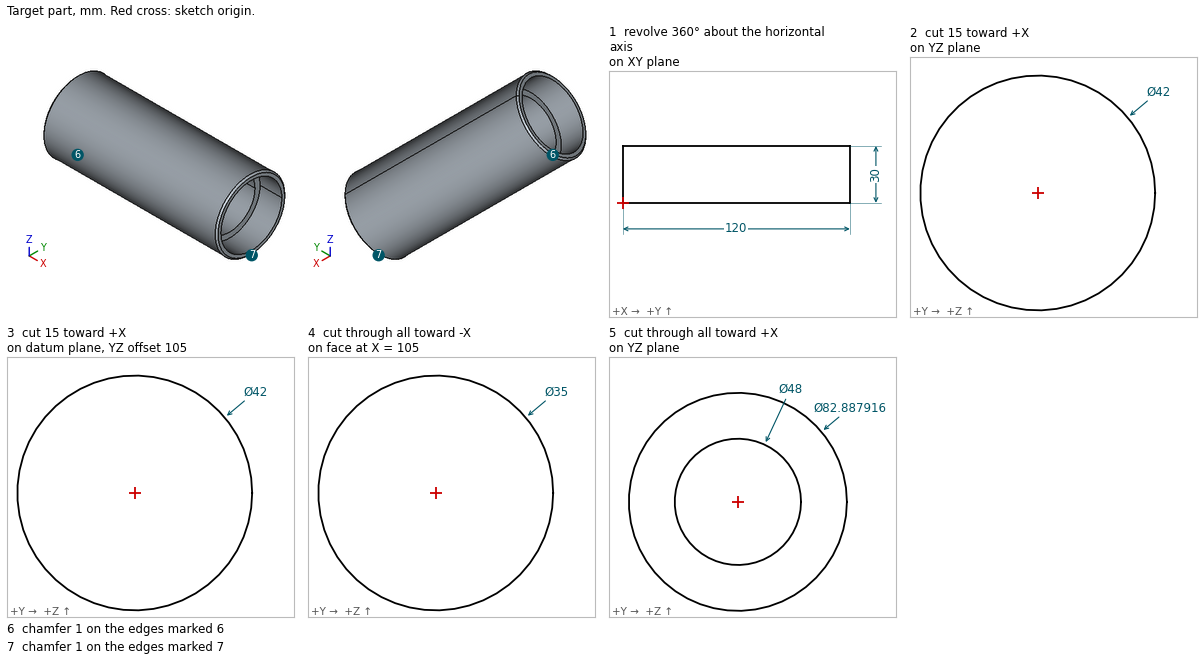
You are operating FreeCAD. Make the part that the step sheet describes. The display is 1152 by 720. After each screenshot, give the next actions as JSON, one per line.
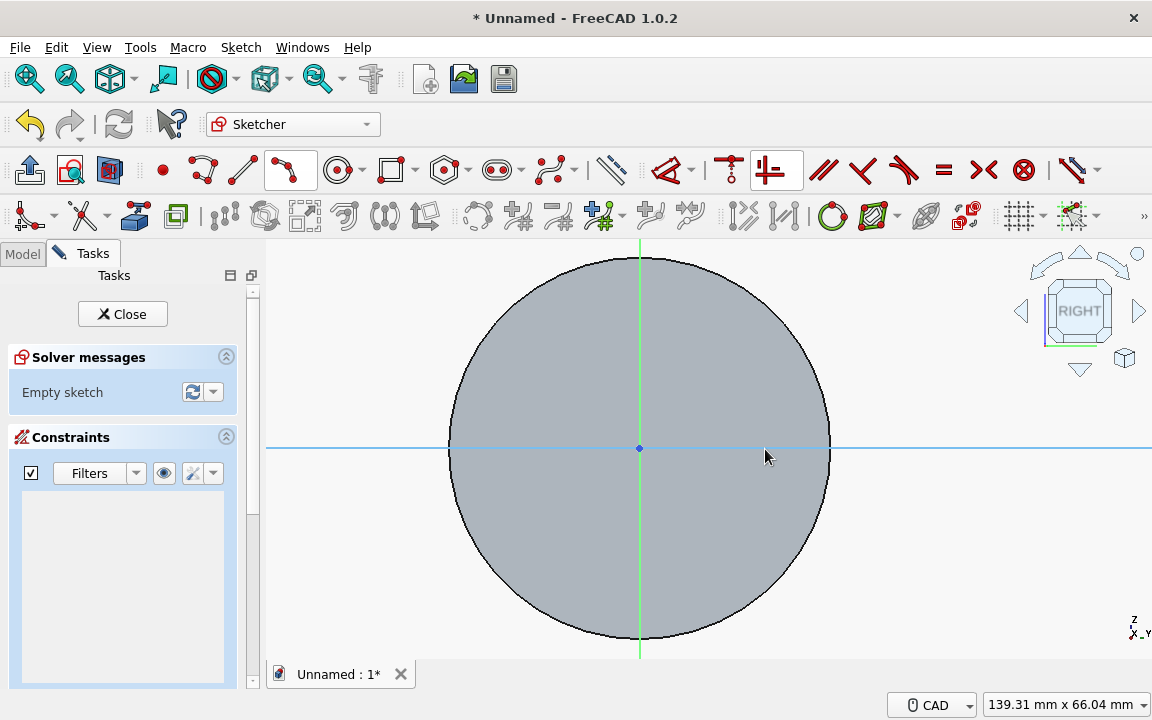
{"action": "key", "text": "g c"}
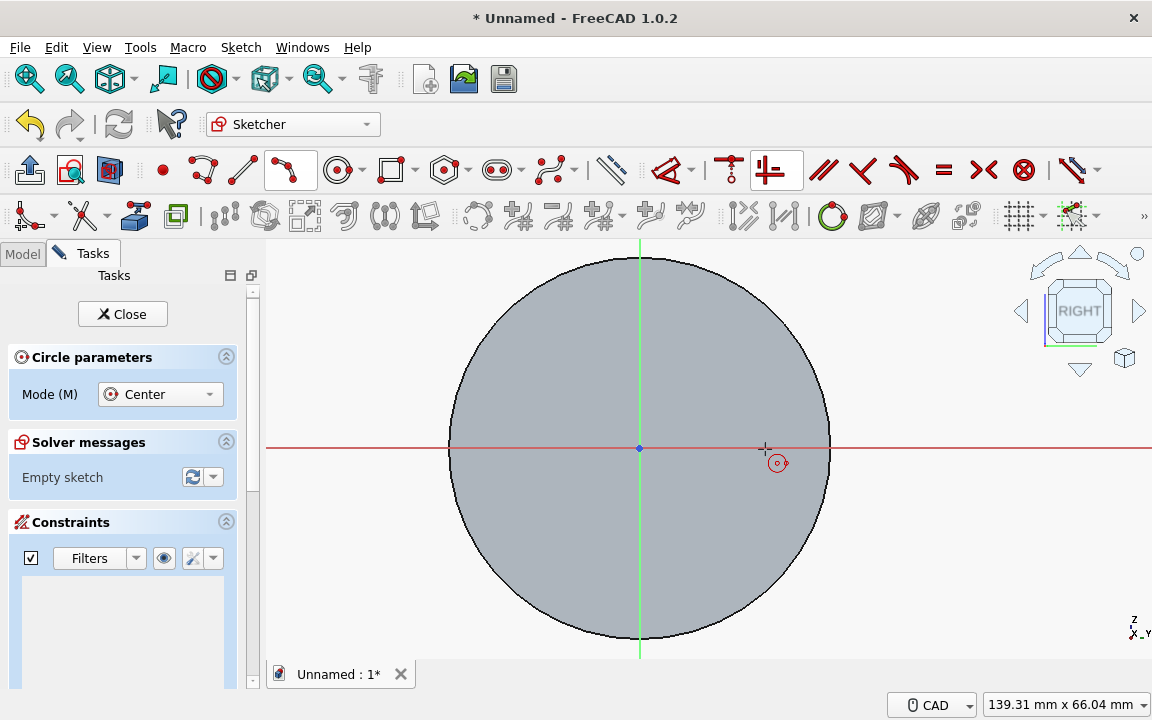
{"action": "left_click", "coordinate": [640, 448]}
{"action": "left_click", "coordinate": [734, 354]}
{"action": "key", "text": "Escape"}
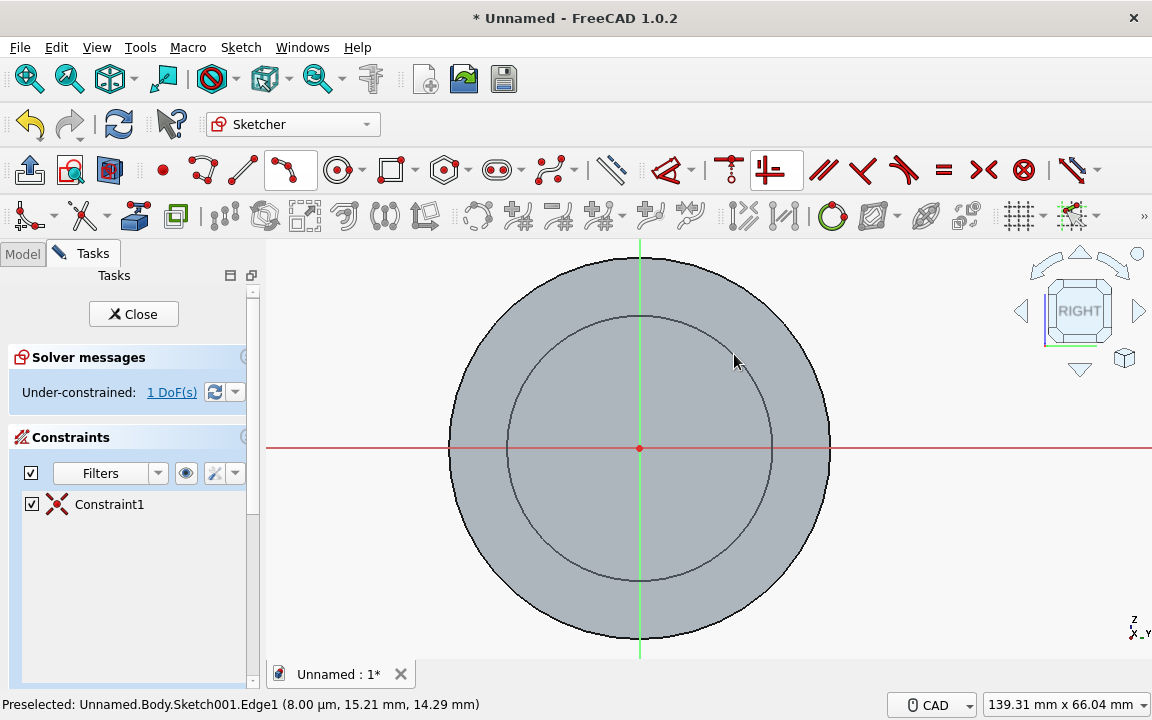
{"action": "left_click", "coordinate": [666, 170]}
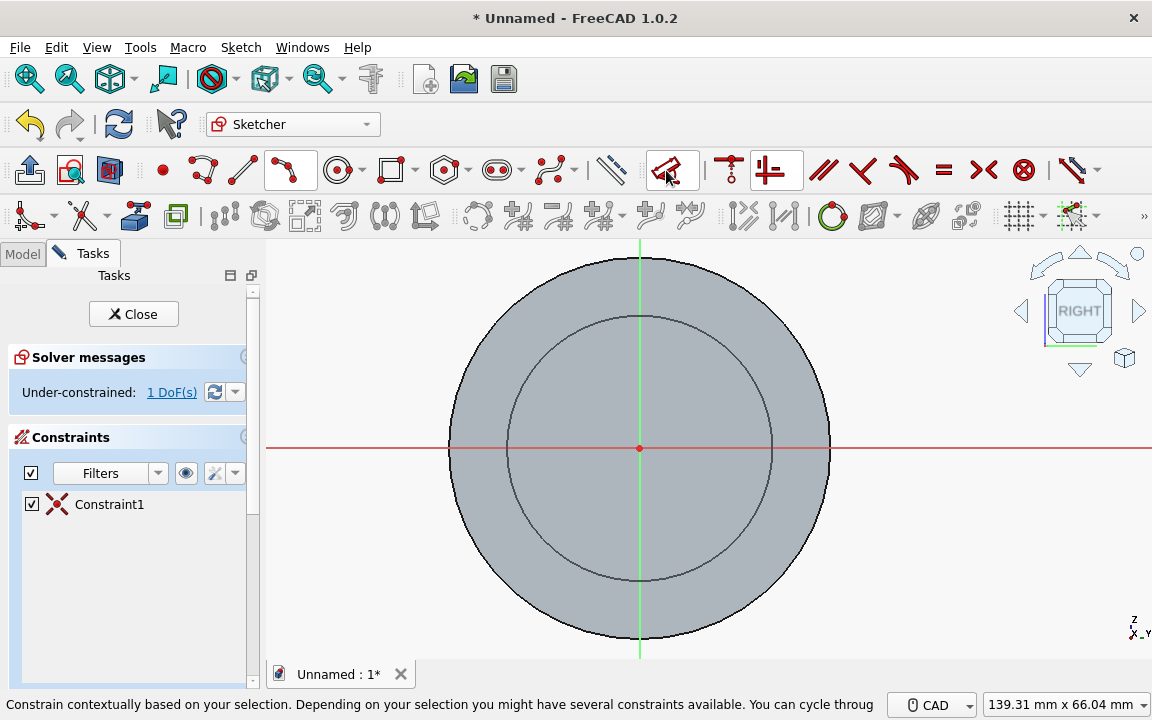
{"action": "left_click", "coordinate": [733, 354]}
{"action": "left_click", "coordinate": [755, 331]}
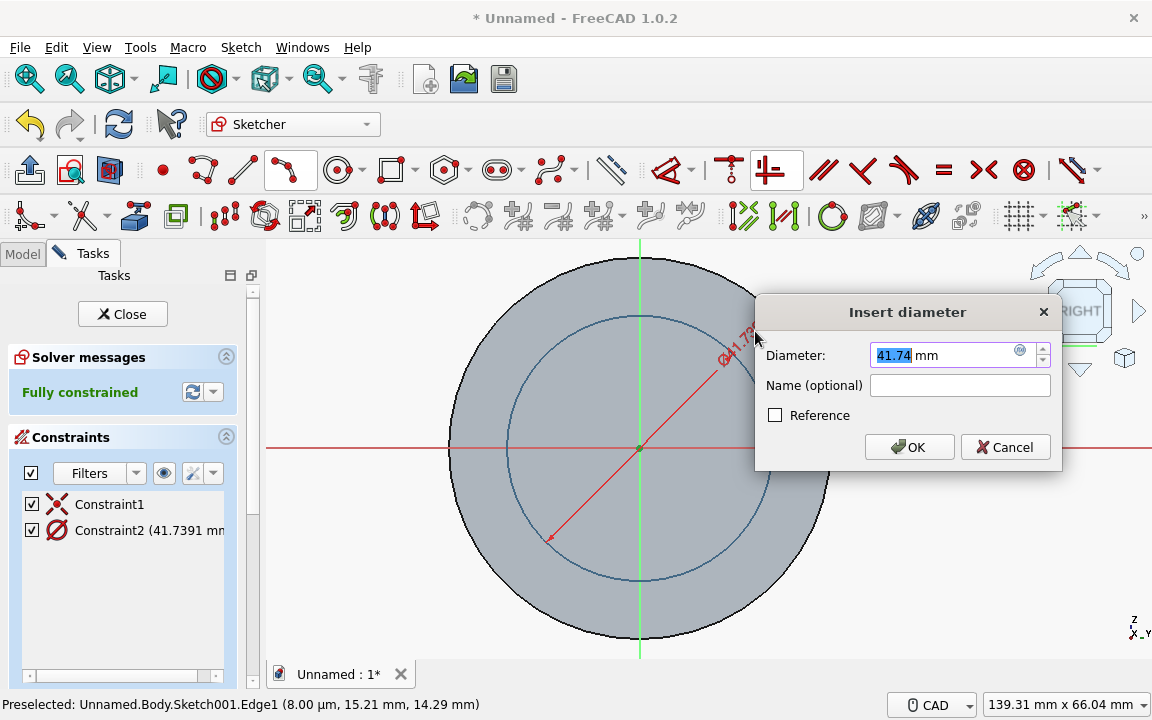
{"action": "type", "text": "42"}
{"action": "key", "text": "Return"}
{"action": "key", "text": "Escape"}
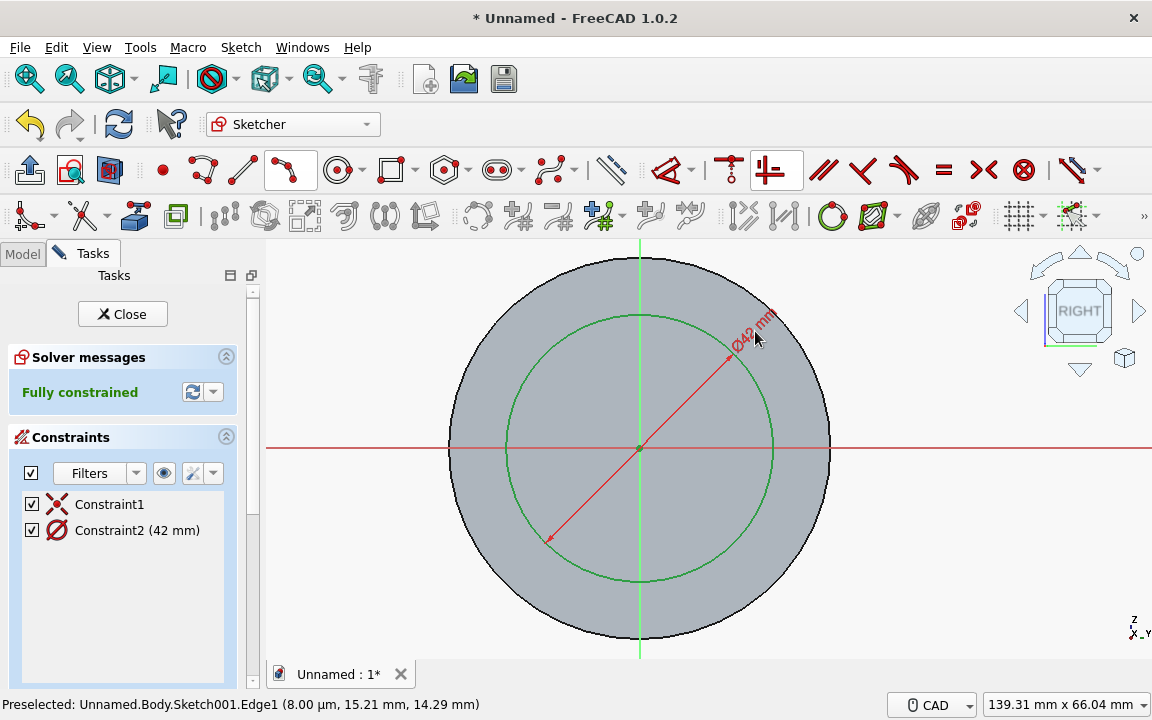
{"action": "left_click", "coordinate": [123, 314]}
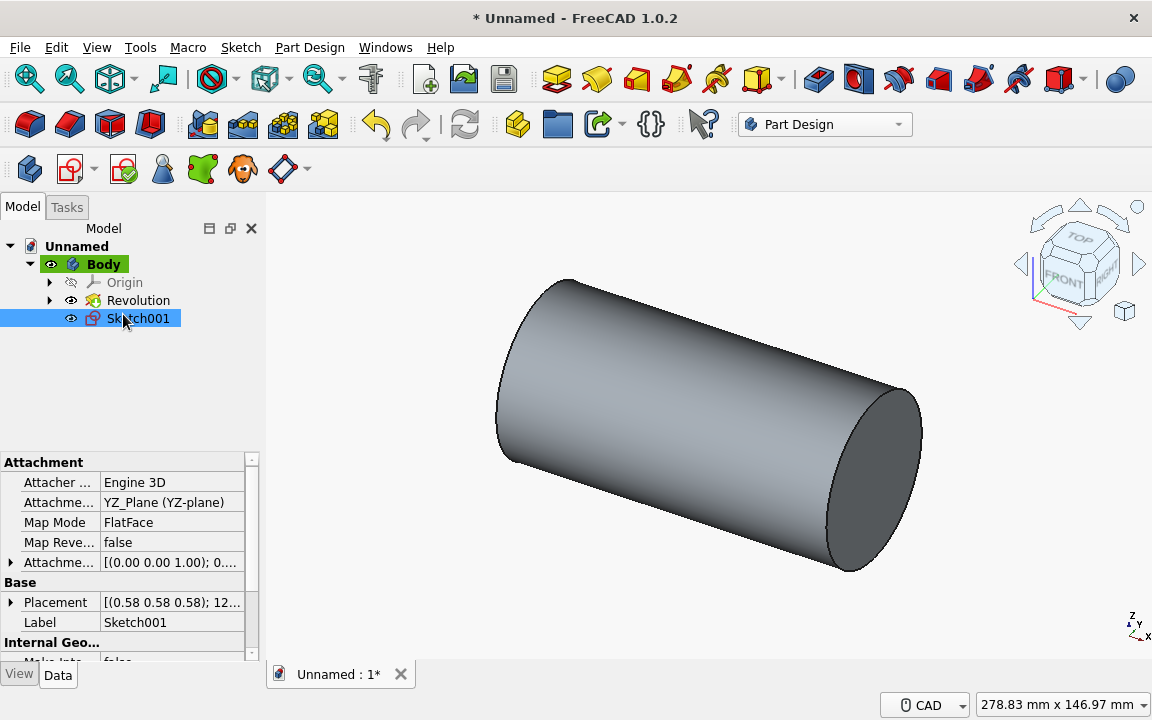
{"action": "left_click", "coordinate": [820, 80]}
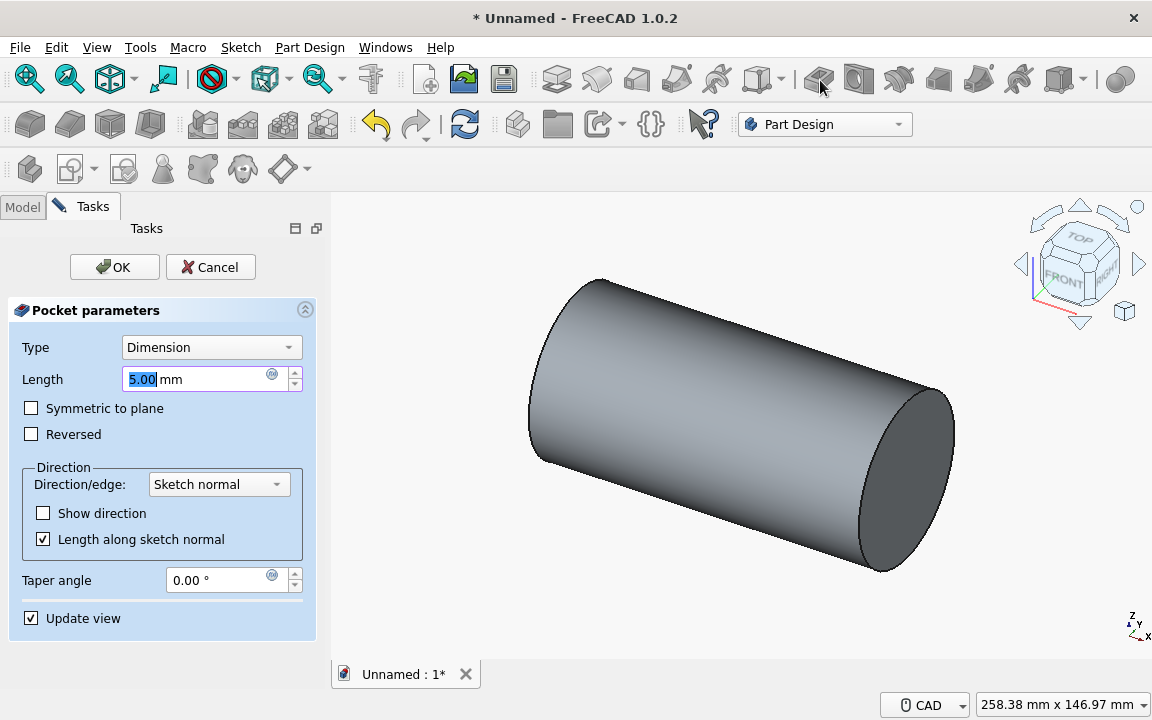
{"action": "type", "text": "15"}
{"action": "key", "text": "Tab"}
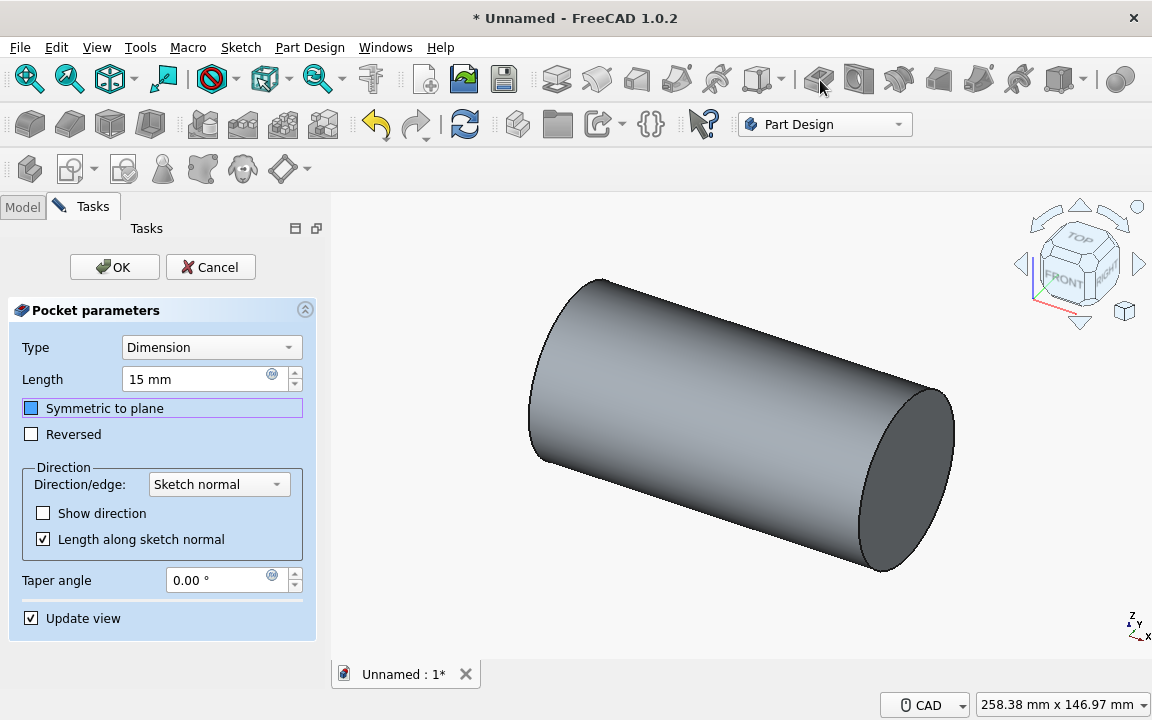
{"action": "left_click", "coordinate": [30, 434]}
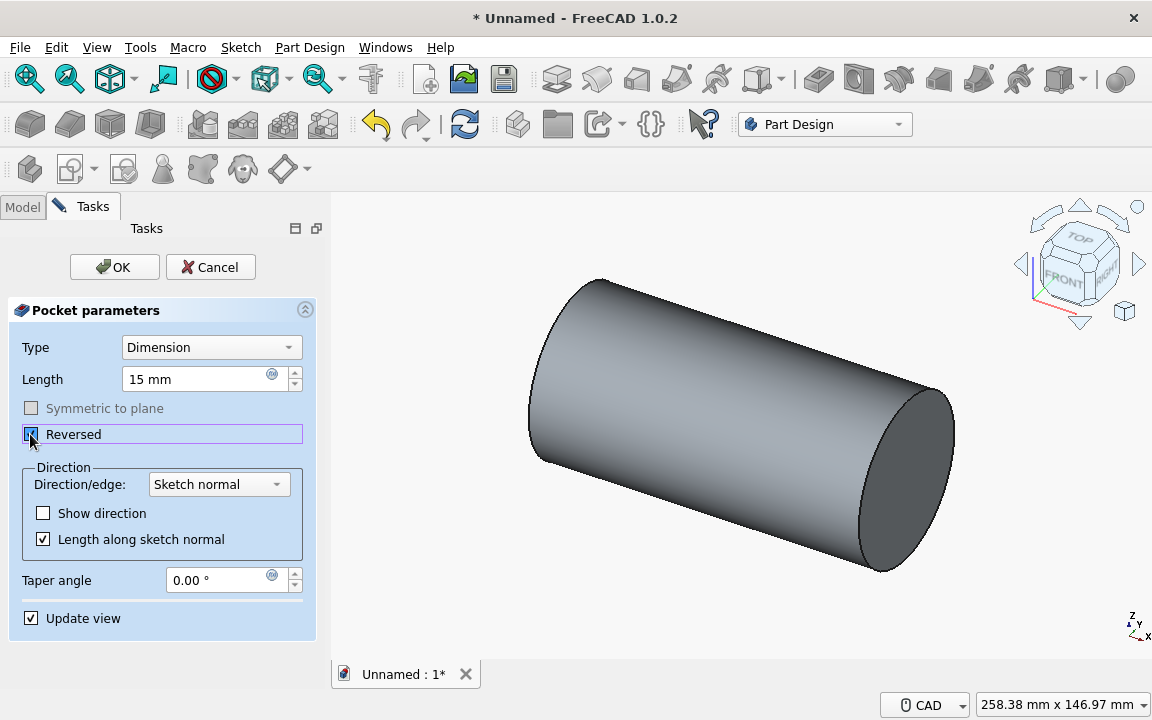
{"action": "left_click", "coordinate": [115, 267]}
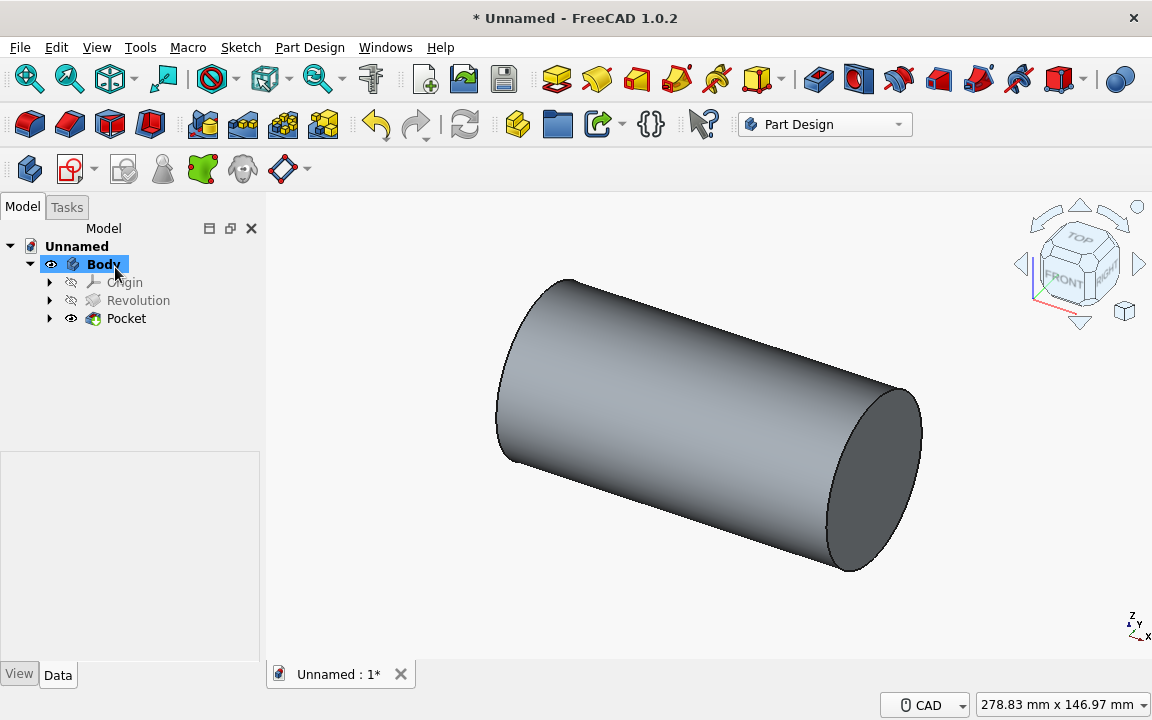
{"action": "left_click", "coordinate": [50, 282]}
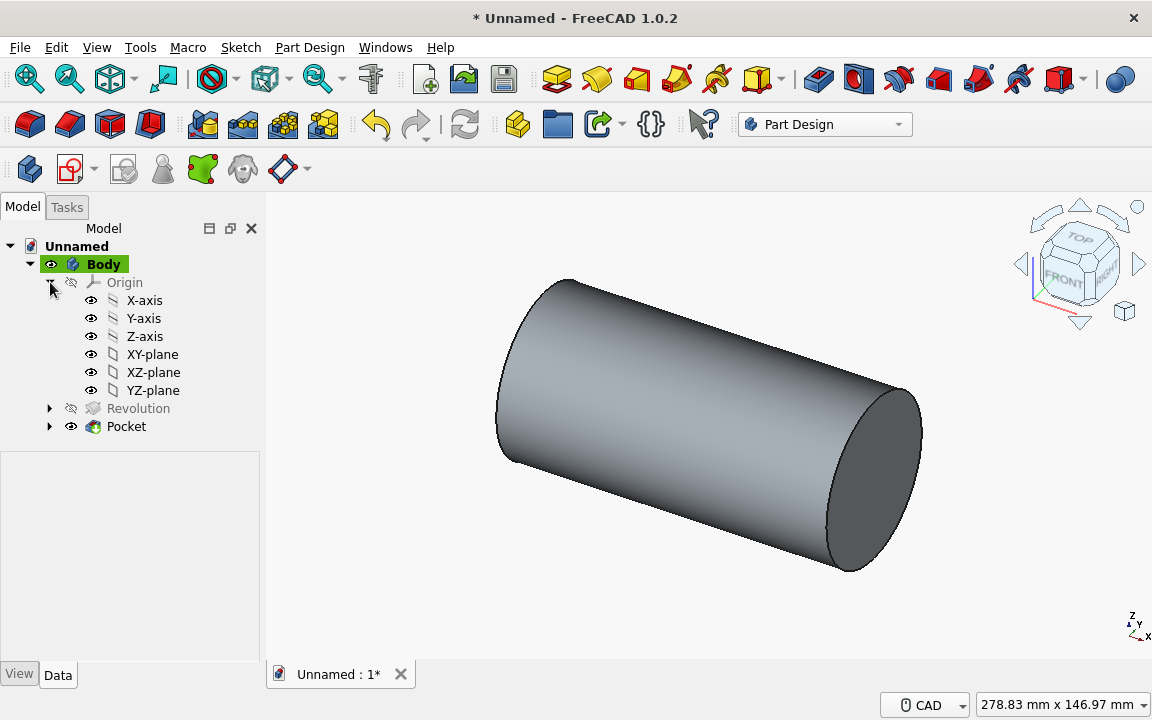
{"action": "left_click", "coordinate": [136, 390]}